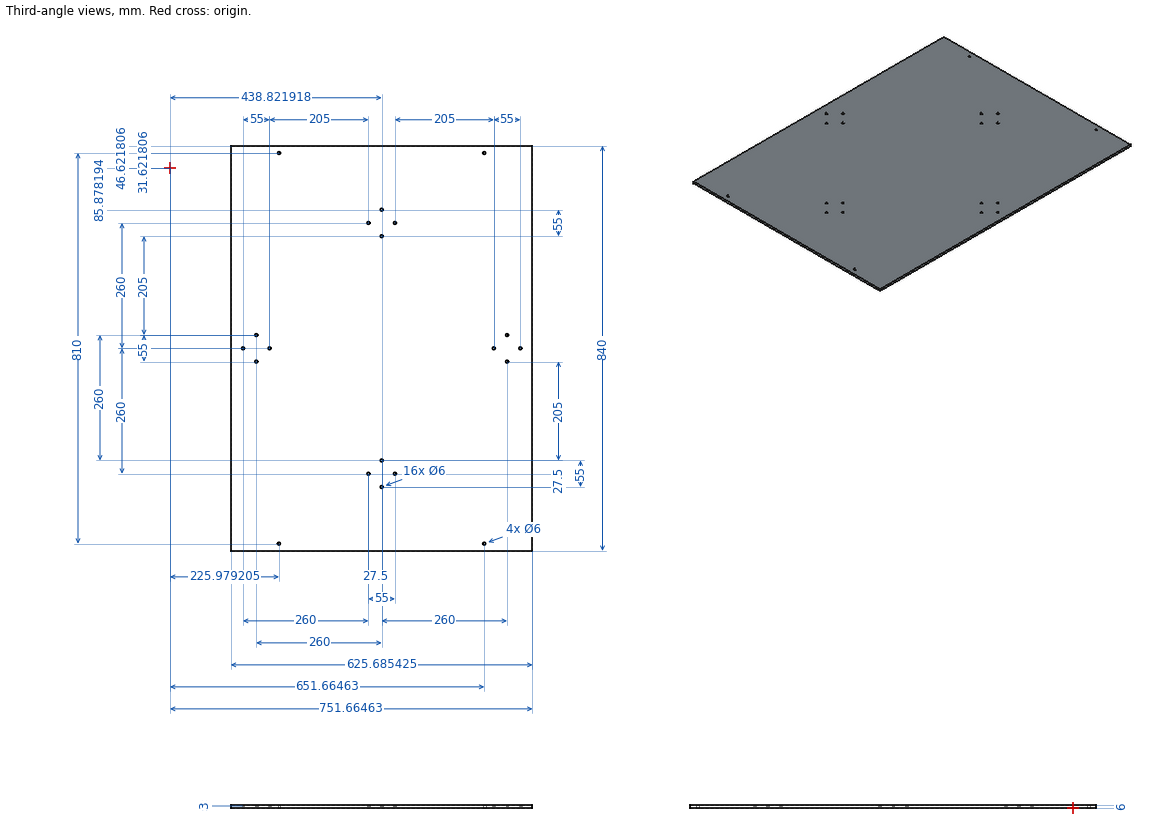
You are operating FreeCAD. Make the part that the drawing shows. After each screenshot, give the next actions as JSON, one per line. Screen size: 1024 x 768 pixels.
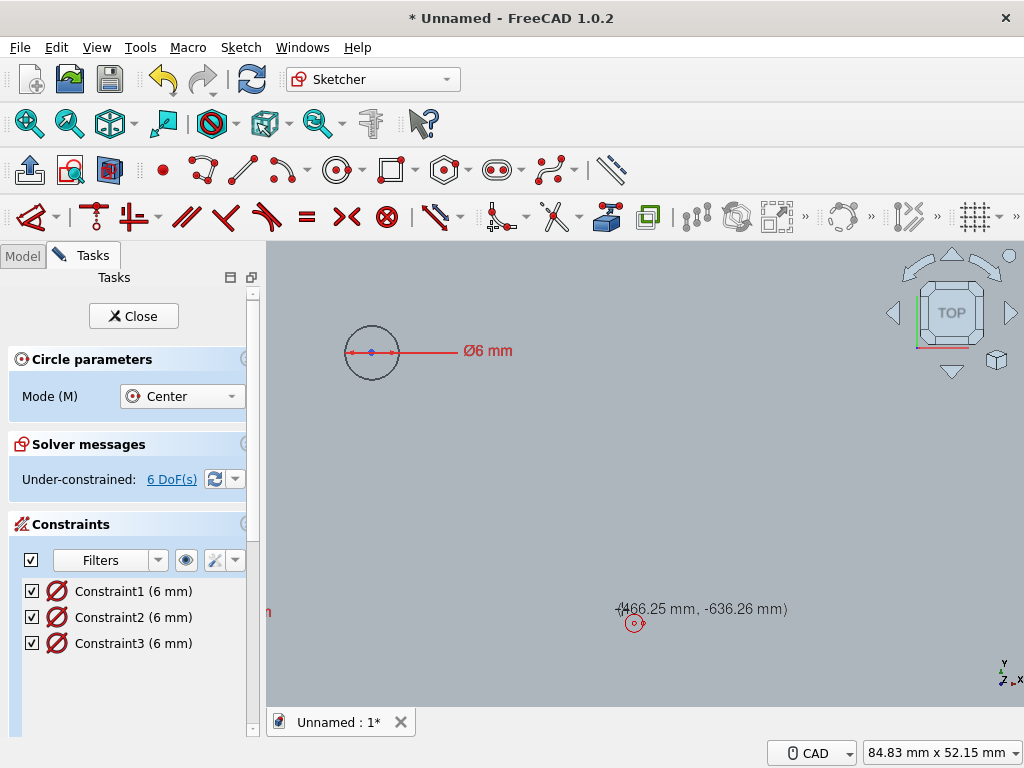
{"action": "scroll", "coordinate": [622, 609], "scroll_direction": "down", "scroll_amount": 15}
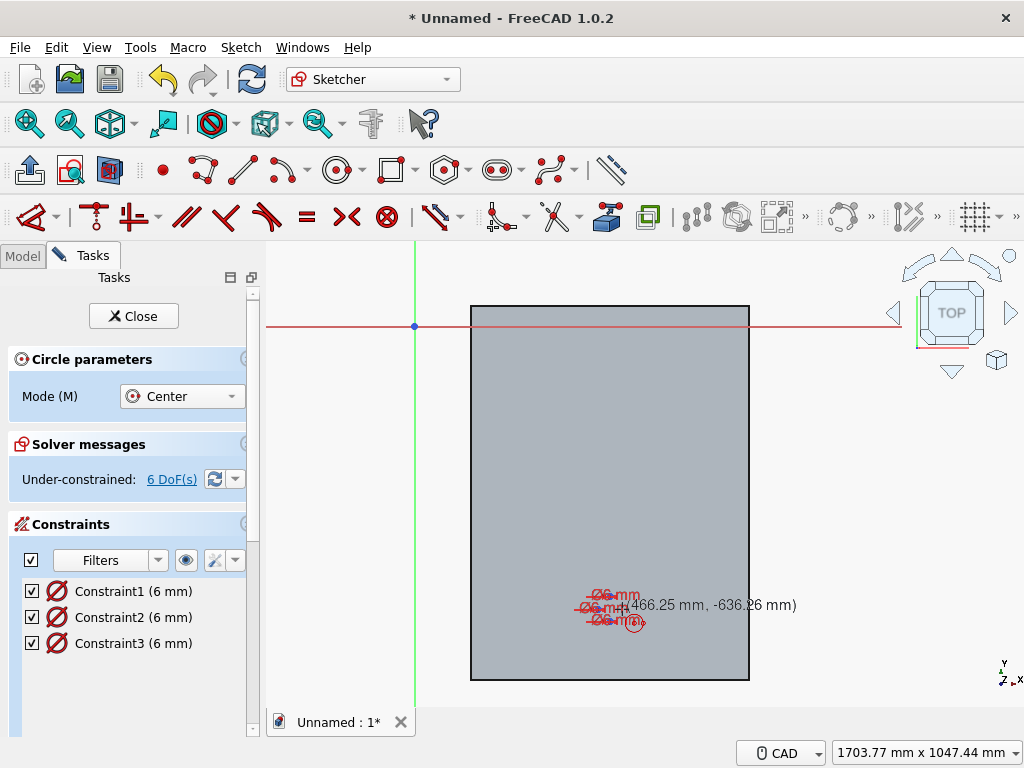
{"action": "left_click", "coordinate": [622, 609]}
{"action": "mouse_move", "coordinate": [623, 608]}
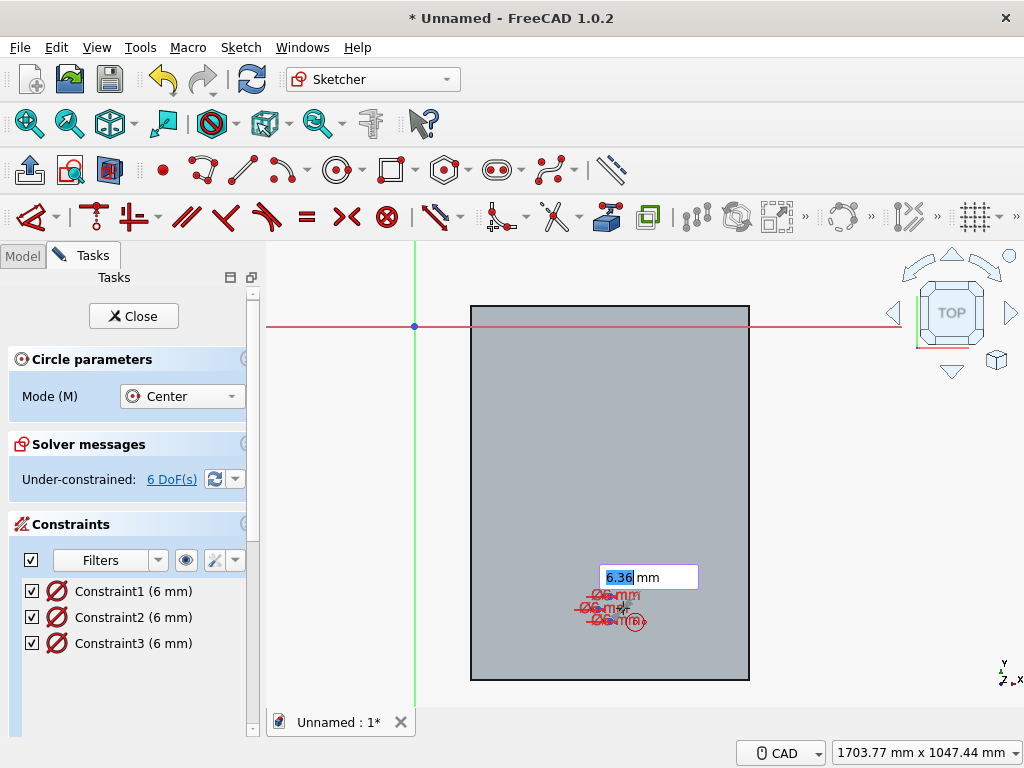
{"action": "type", "text": "6"}
{"action": "key", "text": "Return"}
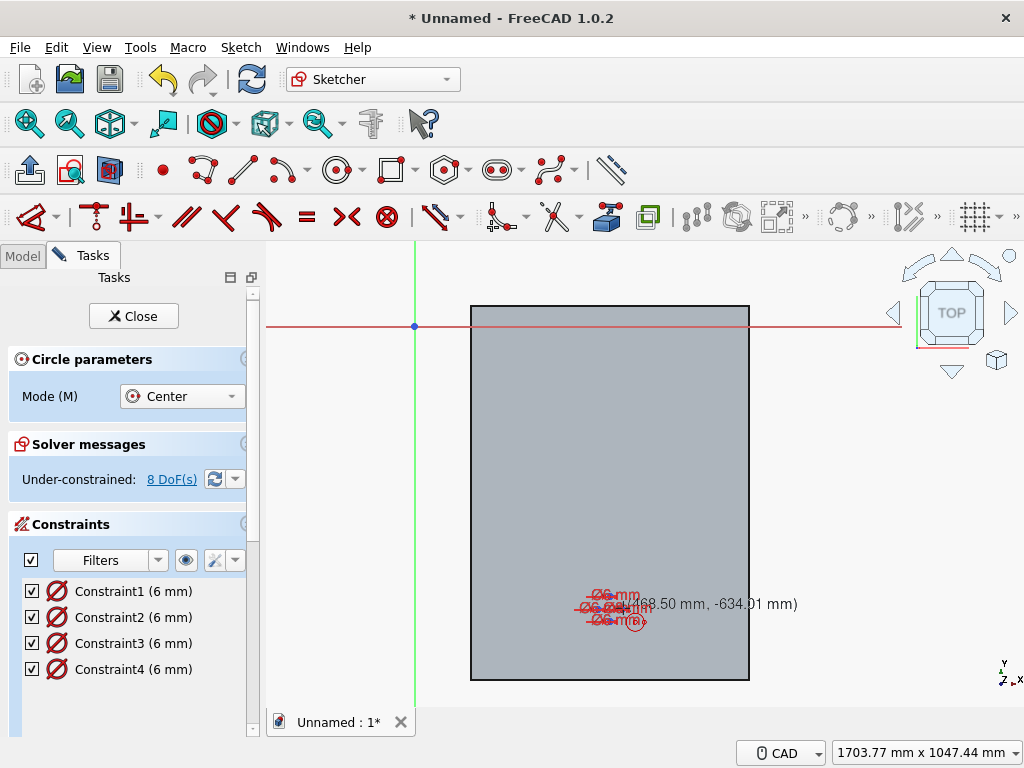
{"action": "scroll", "coordinate": [482, 493], "scroll_direction": "up", "scroll_amount": 15}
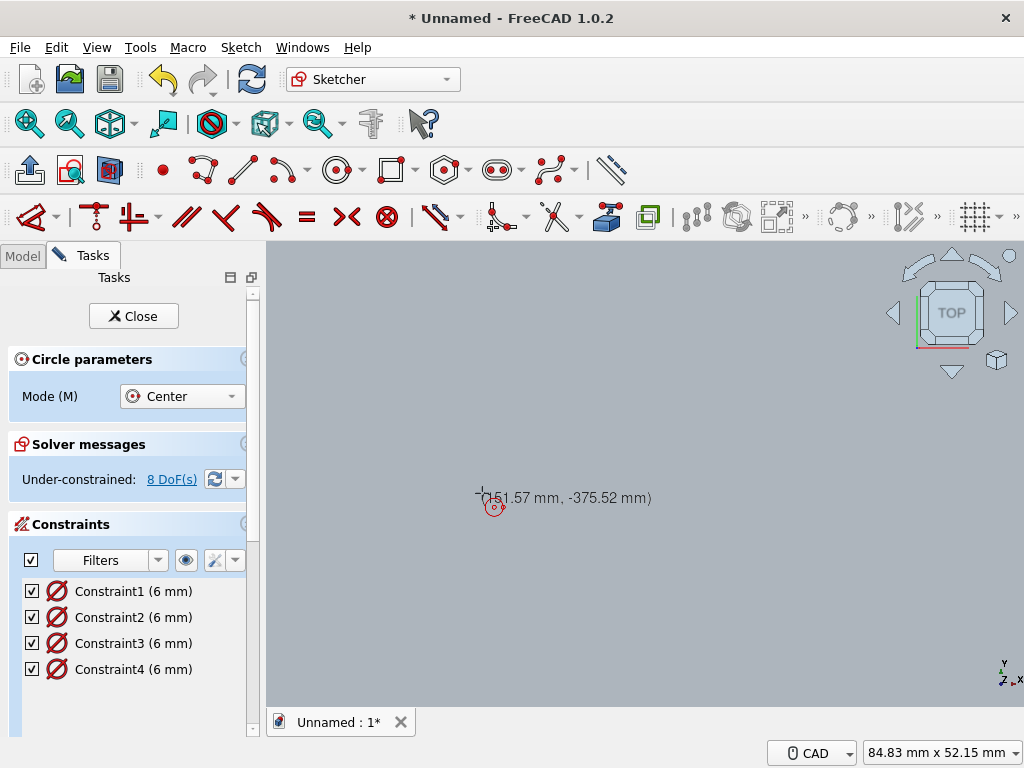
{"action": "scroll", "coordinate": [482, 493], "scroll_direction": "down", "scroll_amount": 15}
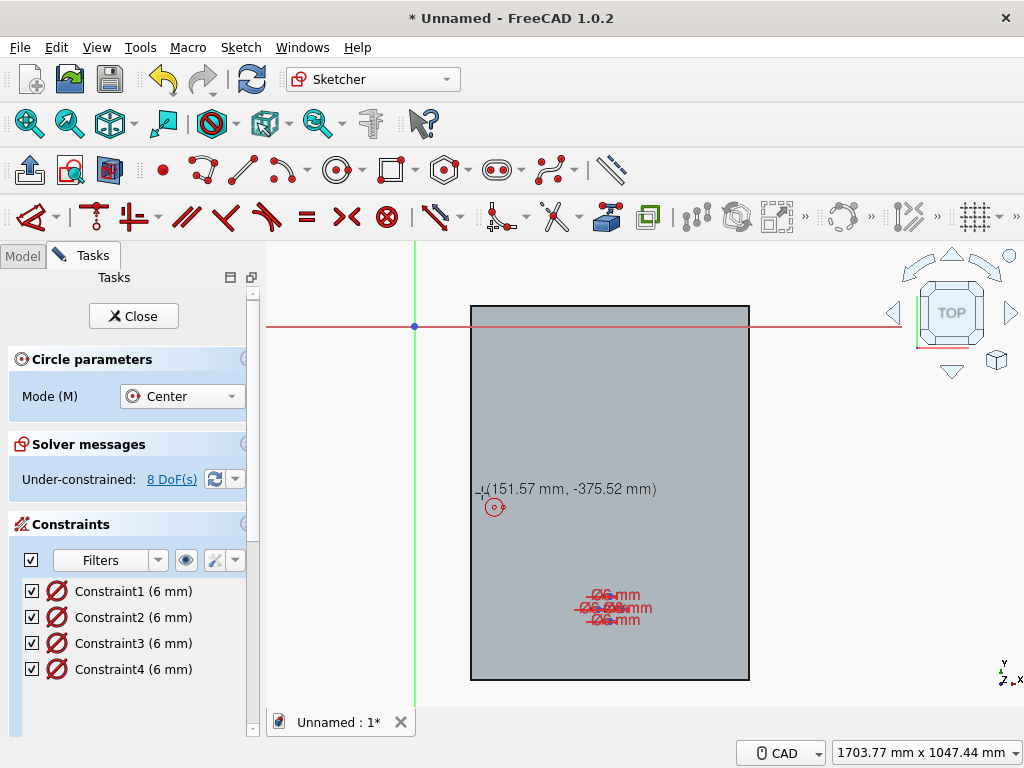
{"action": "left_click", "coordinate": [482, 493]}
{"action": "mouse_move", "coordinate": [483, 492]}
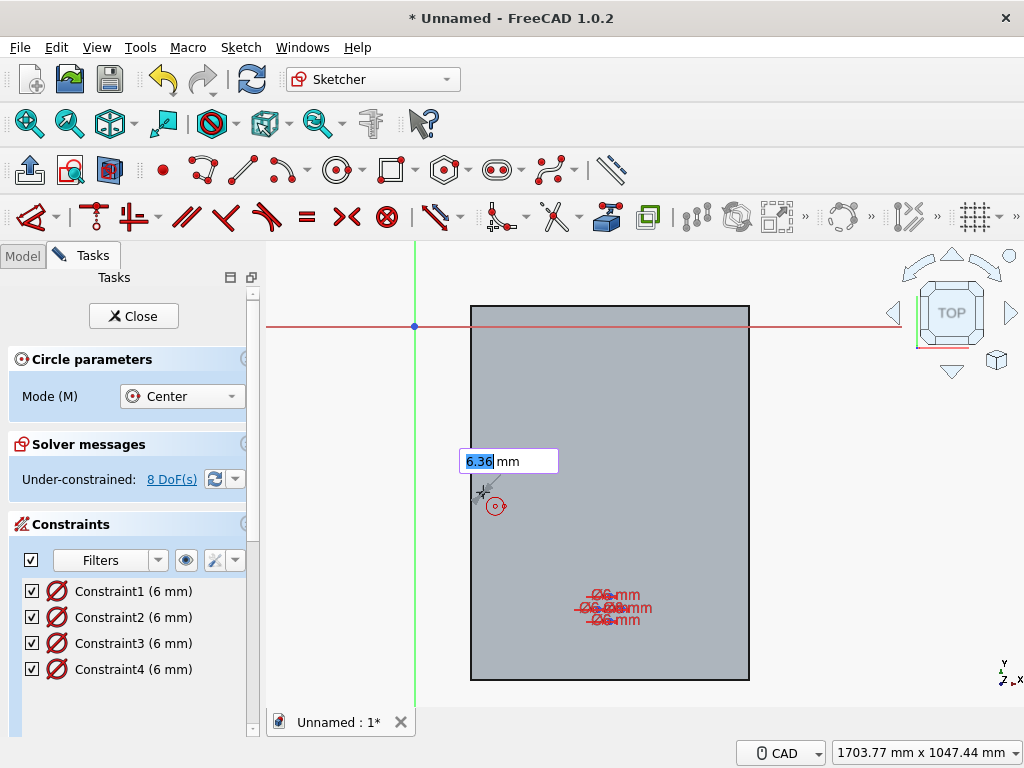
{"action": "type", "text": "6"}
{"action": "key", "text": "Return"}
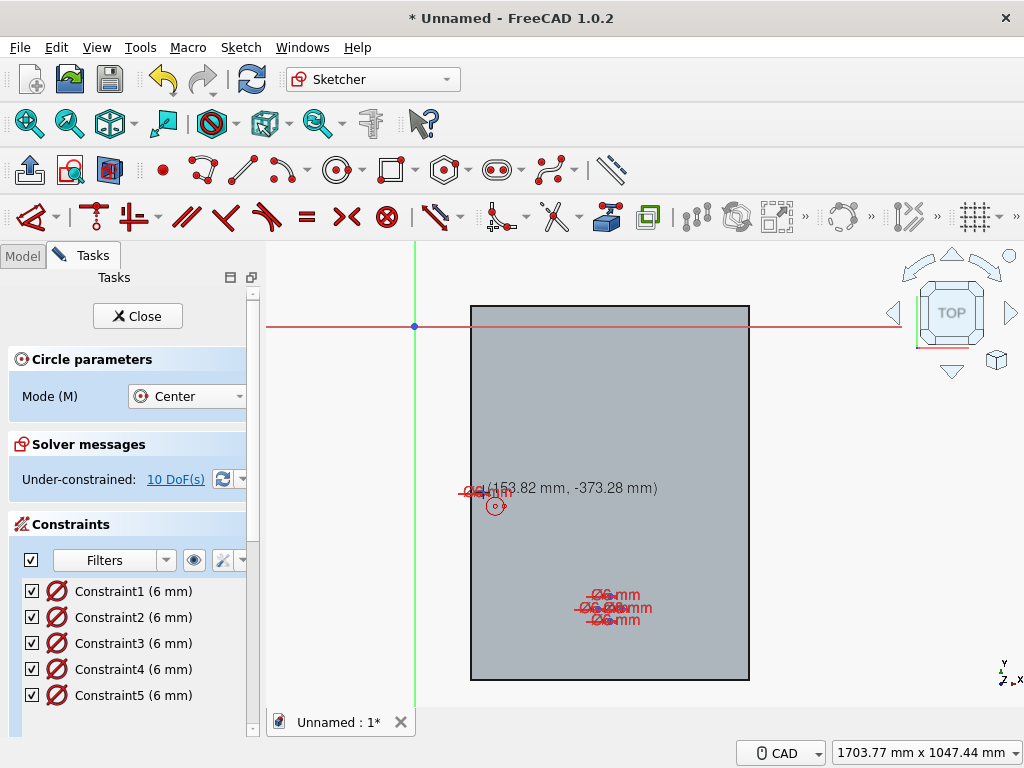
{"action": "scroll", "coordinate": [494, 481], "scroll_direction": "up", "scroll_amount": 15}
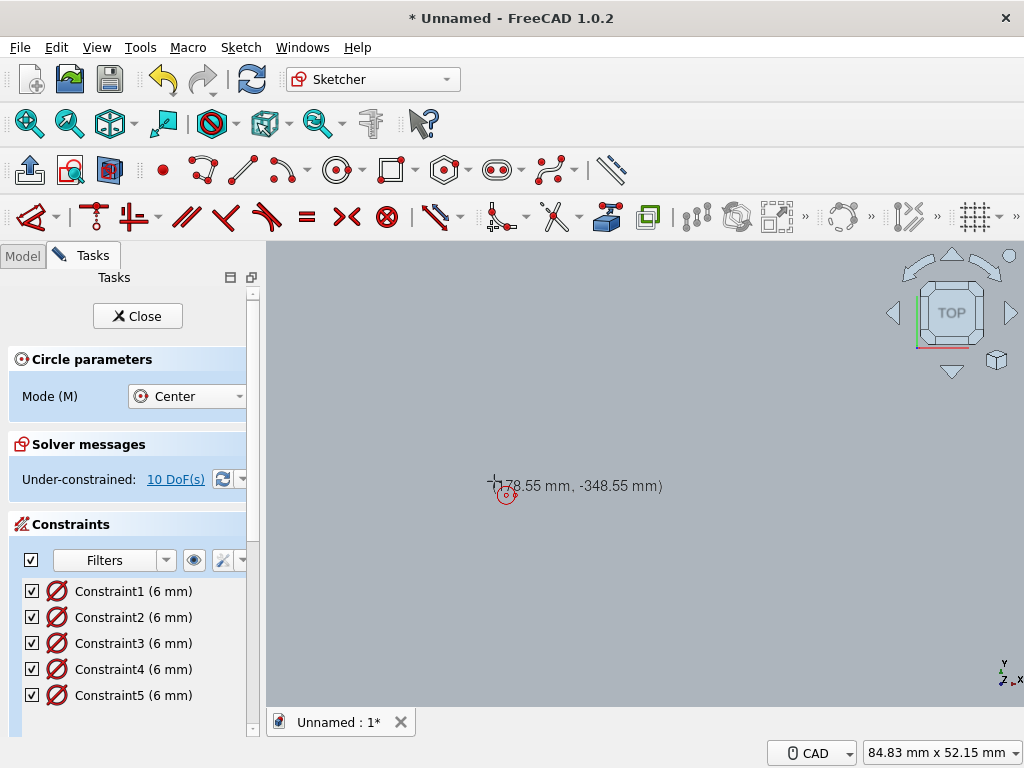
{"action": "scroll", "coordinate": [494, 481], "scroll_direction": "down", "scroll_amount": 15}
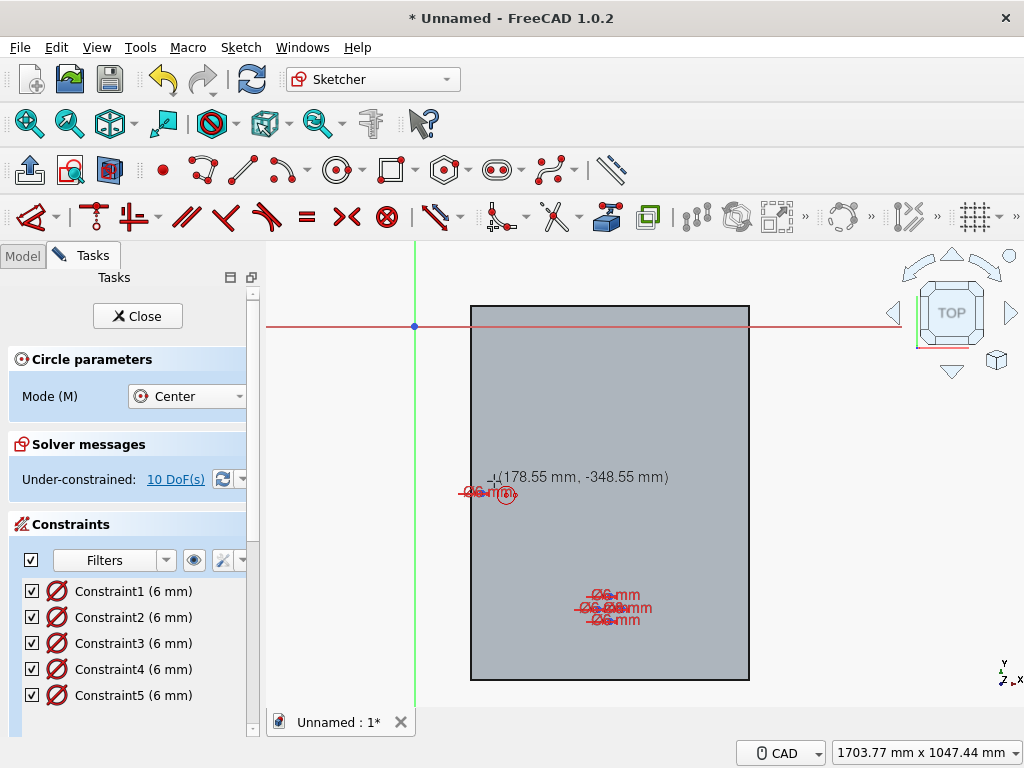
{"action": "left_click", "coordinate": [494, 481]}
{"action": "mouse_move", "coordinate": [495, 480]}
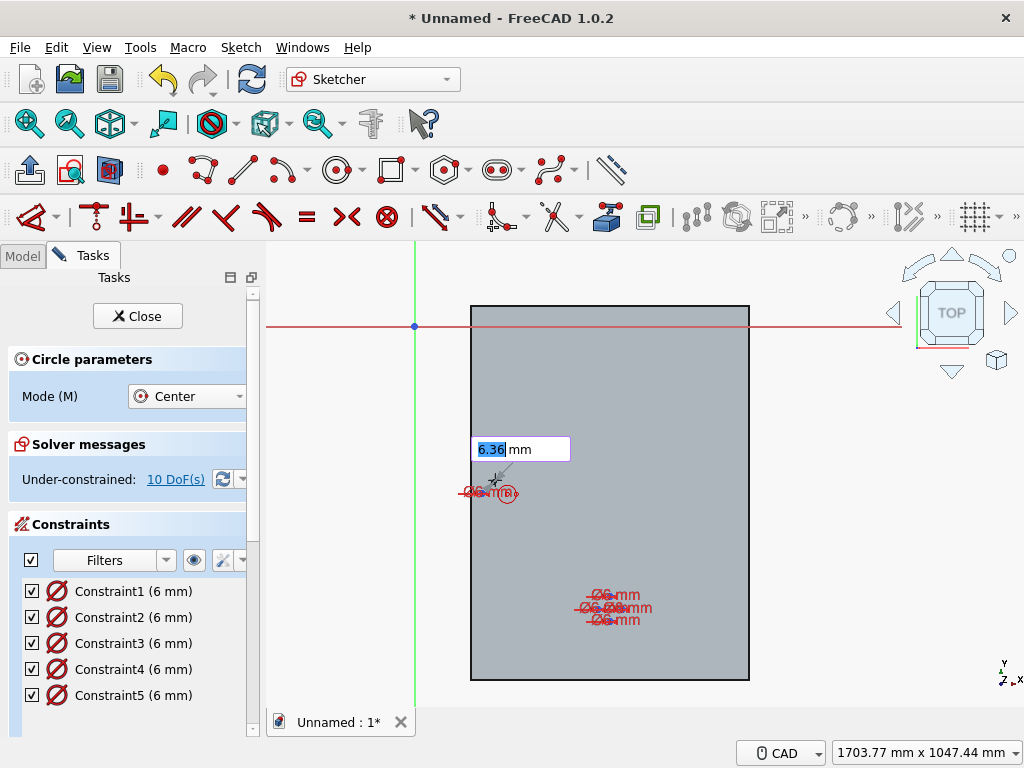
{"action": "type", "text": "6"}
{"action": "key", "text": "Return"}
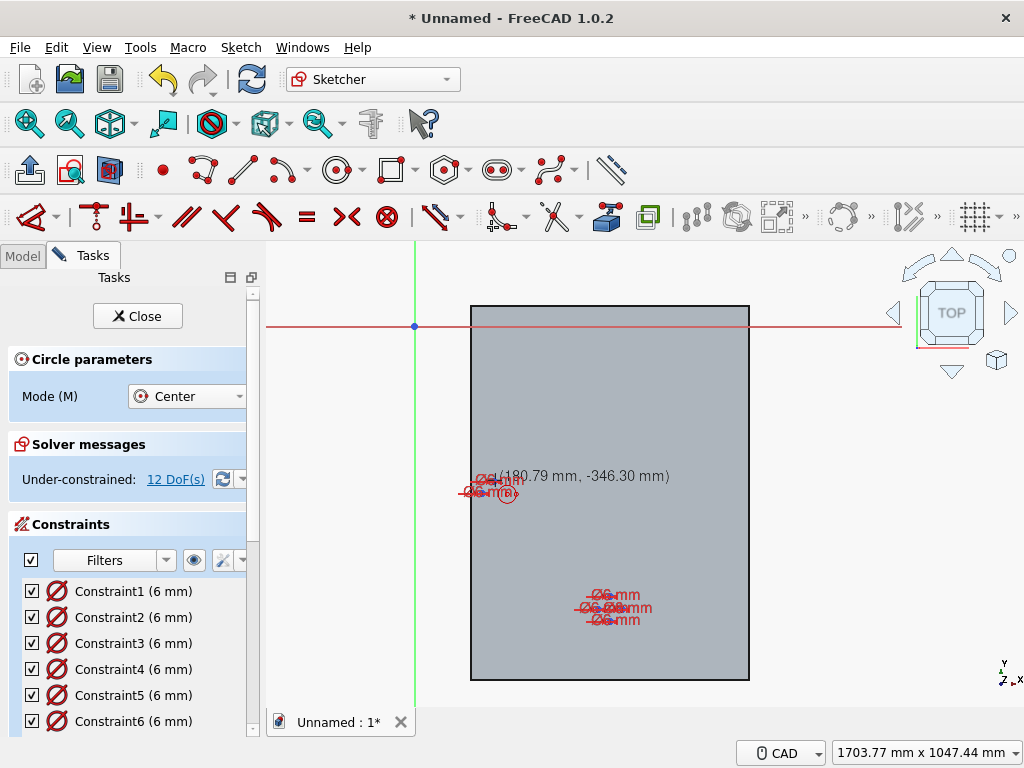
{"action": "scroll", "coordinate": [506, 493], "scroll_direction": "up", "scroll_amount": 15}